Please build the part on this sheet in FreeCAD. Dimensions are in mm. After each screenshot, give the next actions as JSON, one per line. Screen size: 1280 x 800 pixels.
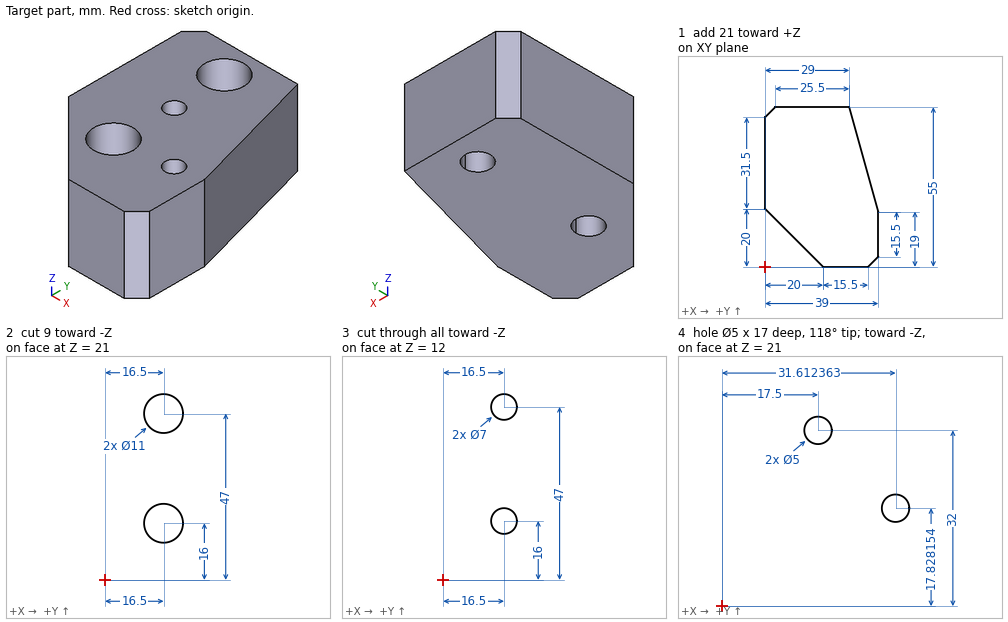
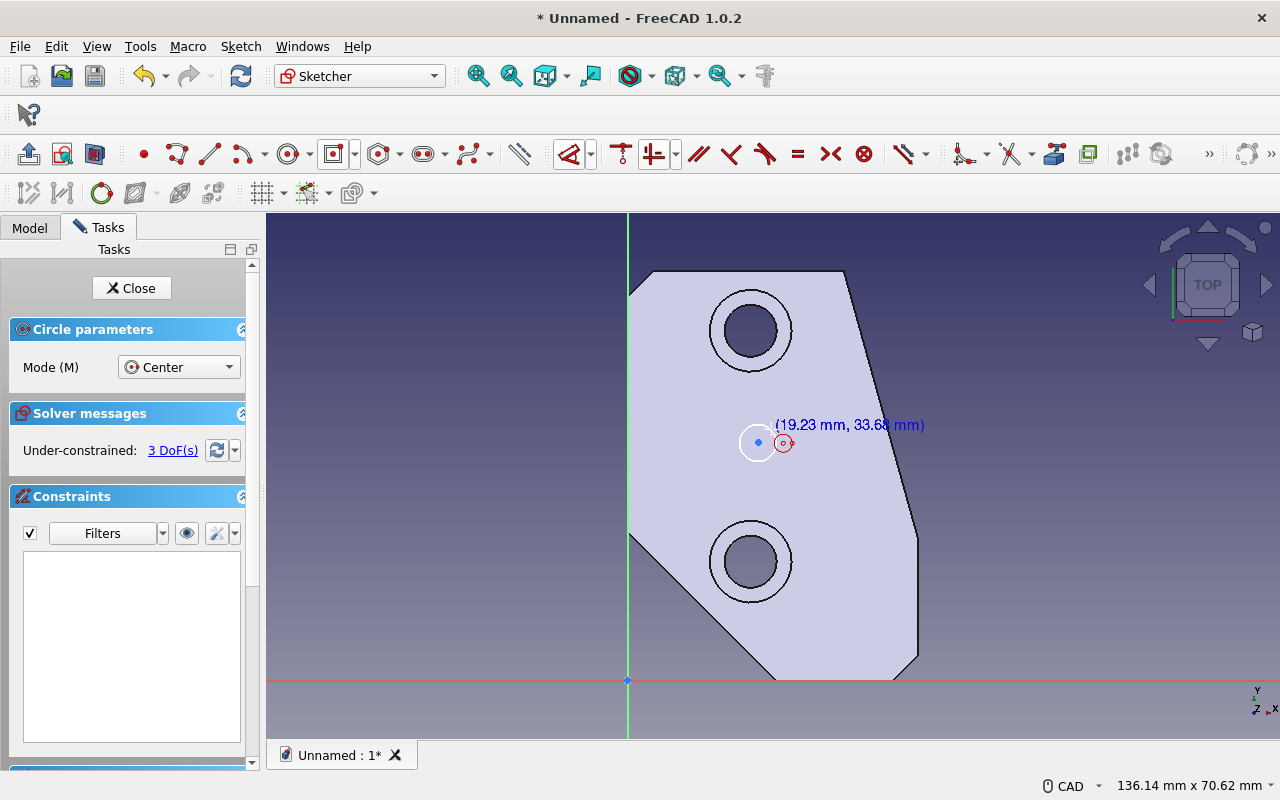
{"action": "left_click", "coordinate": [863, 548]}
{"action": "left_click", "coordinate": [876, 535]}
{"action": "key", "text": "Escape"}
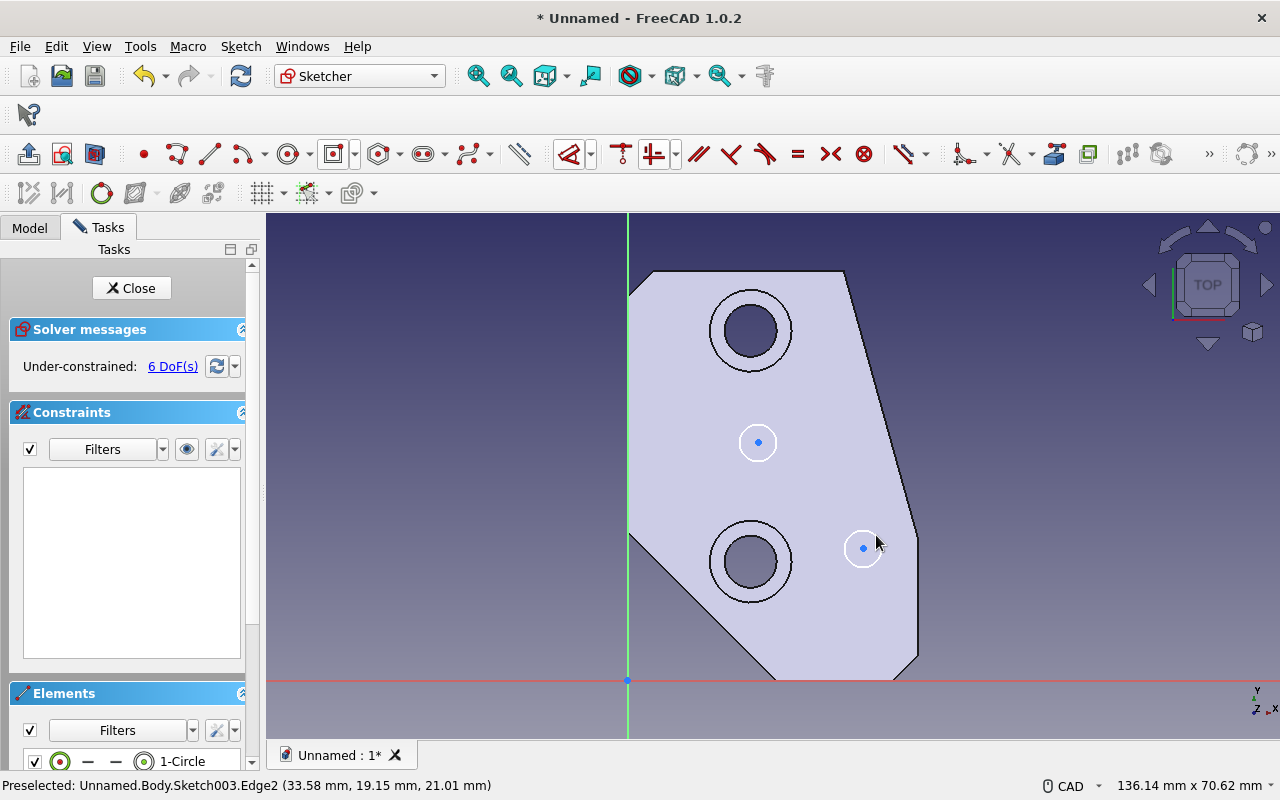
{"action": "left_click", "coordinate": [771, 430]}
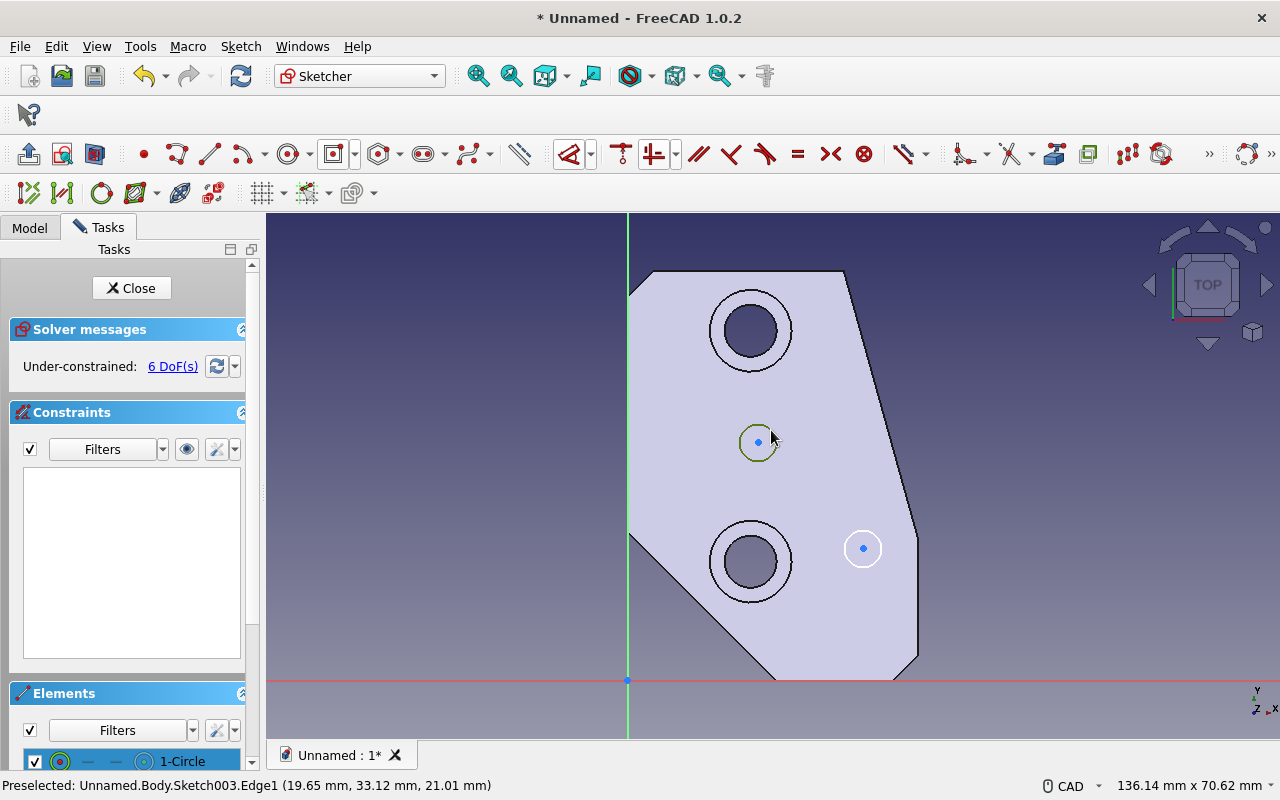
{"action": "left_click", "coordinate": [876, 536]}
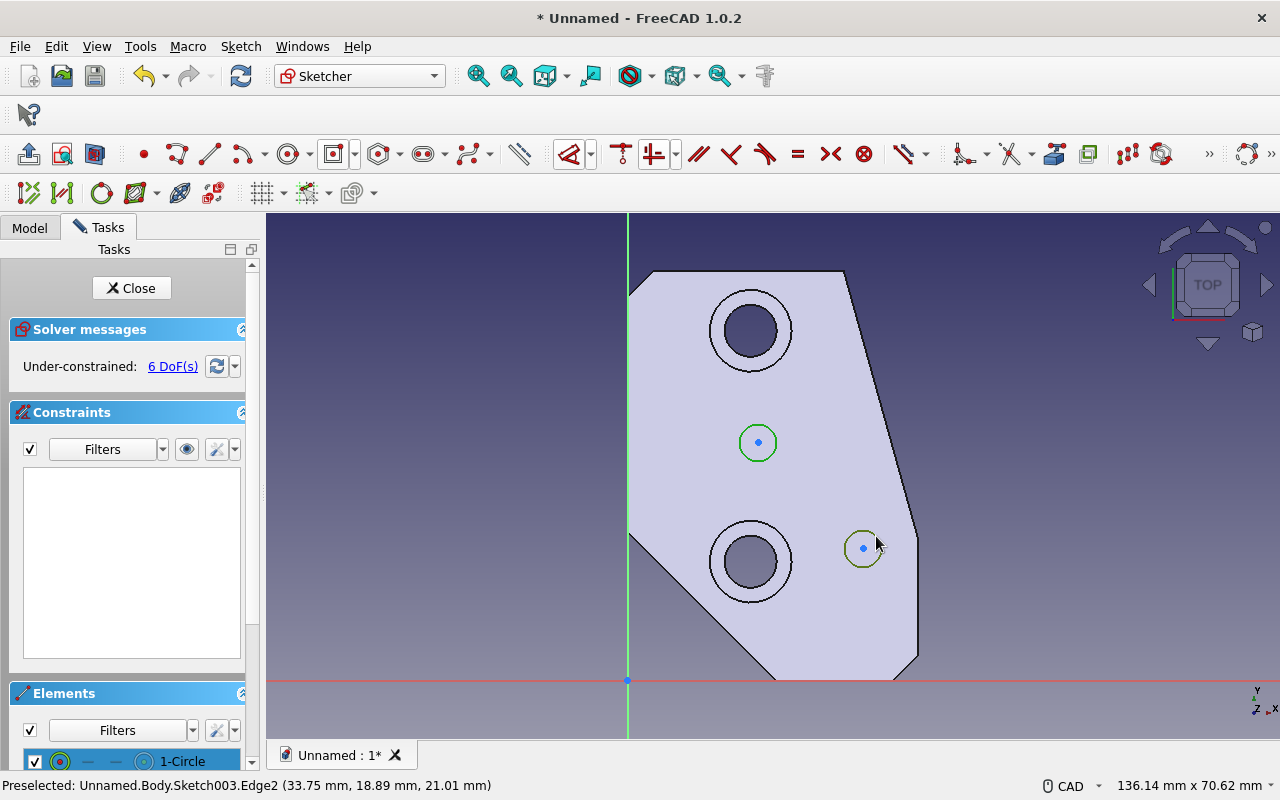
{"action": "left_click", "coordinate": [798, 154]}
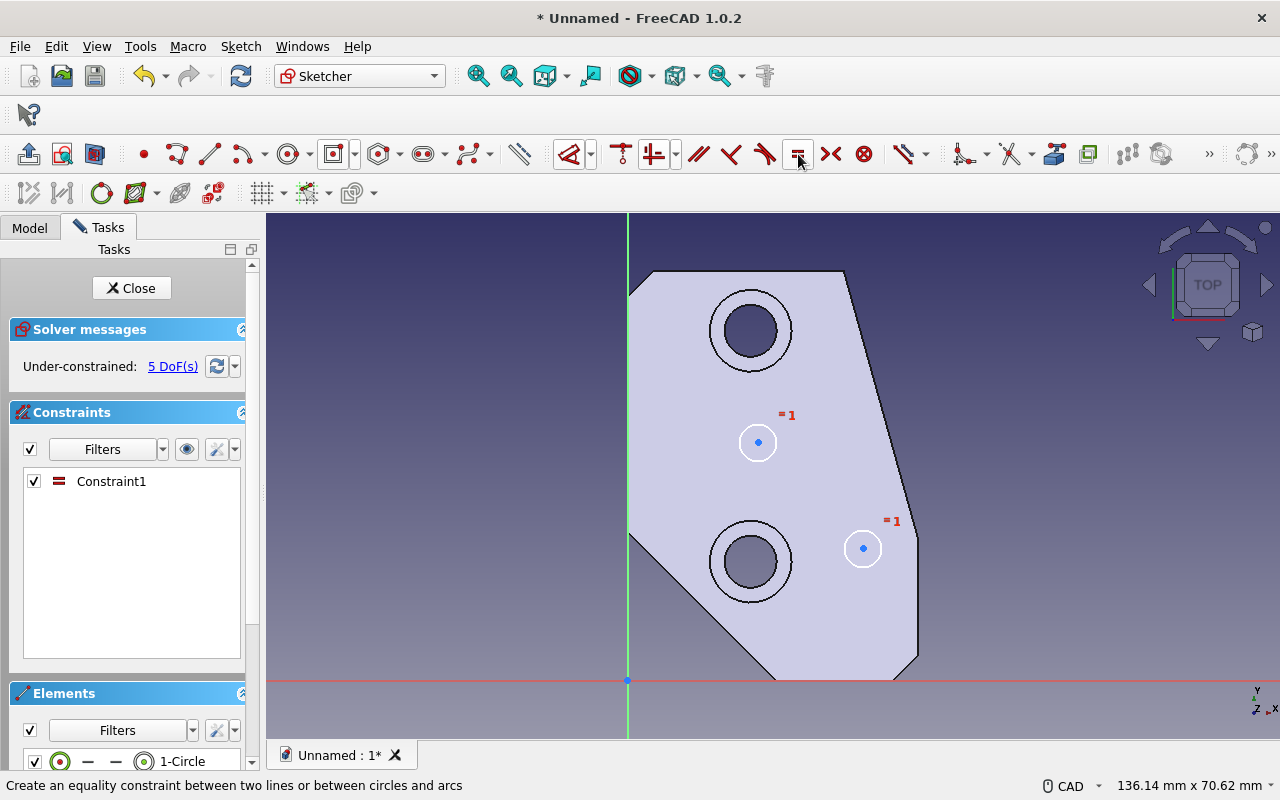
{"action": "left_click", "coordinate": [771, 430]}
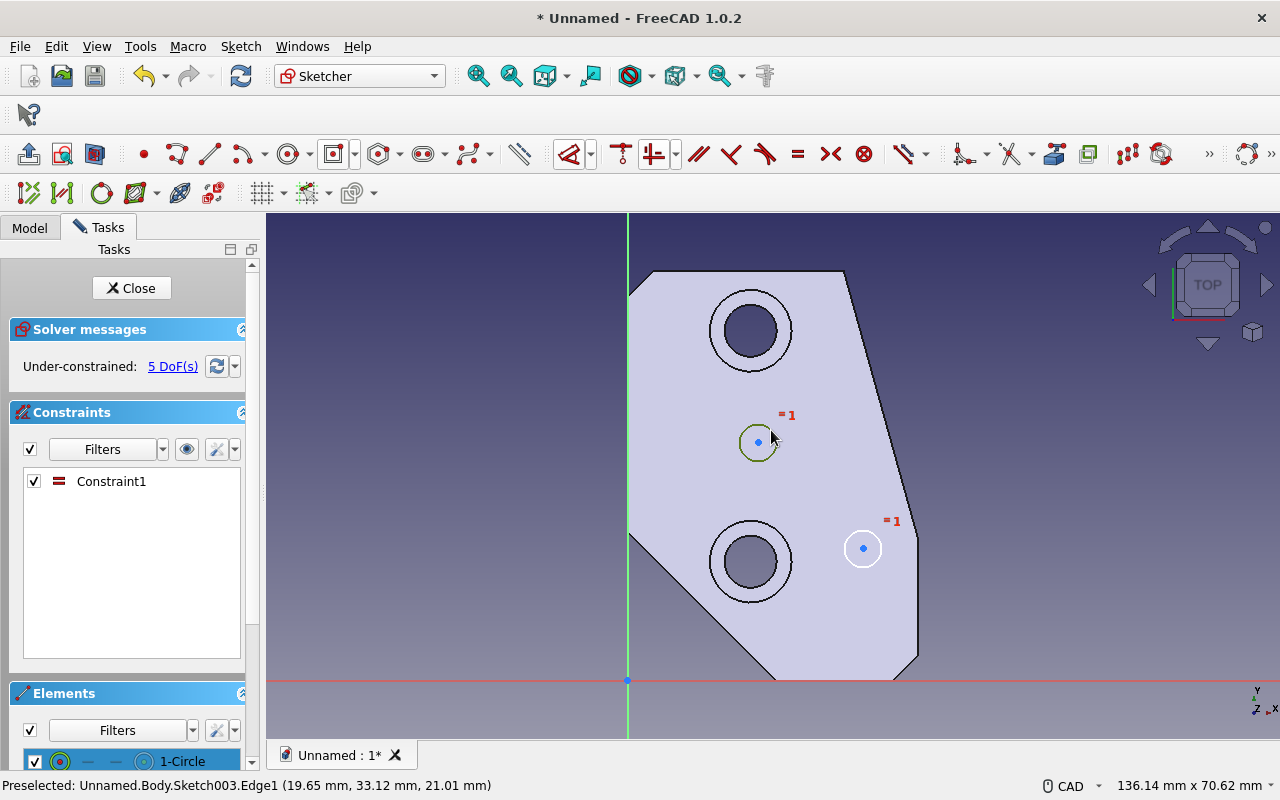
{"action": "left_click", "coordinate": [590, 154]}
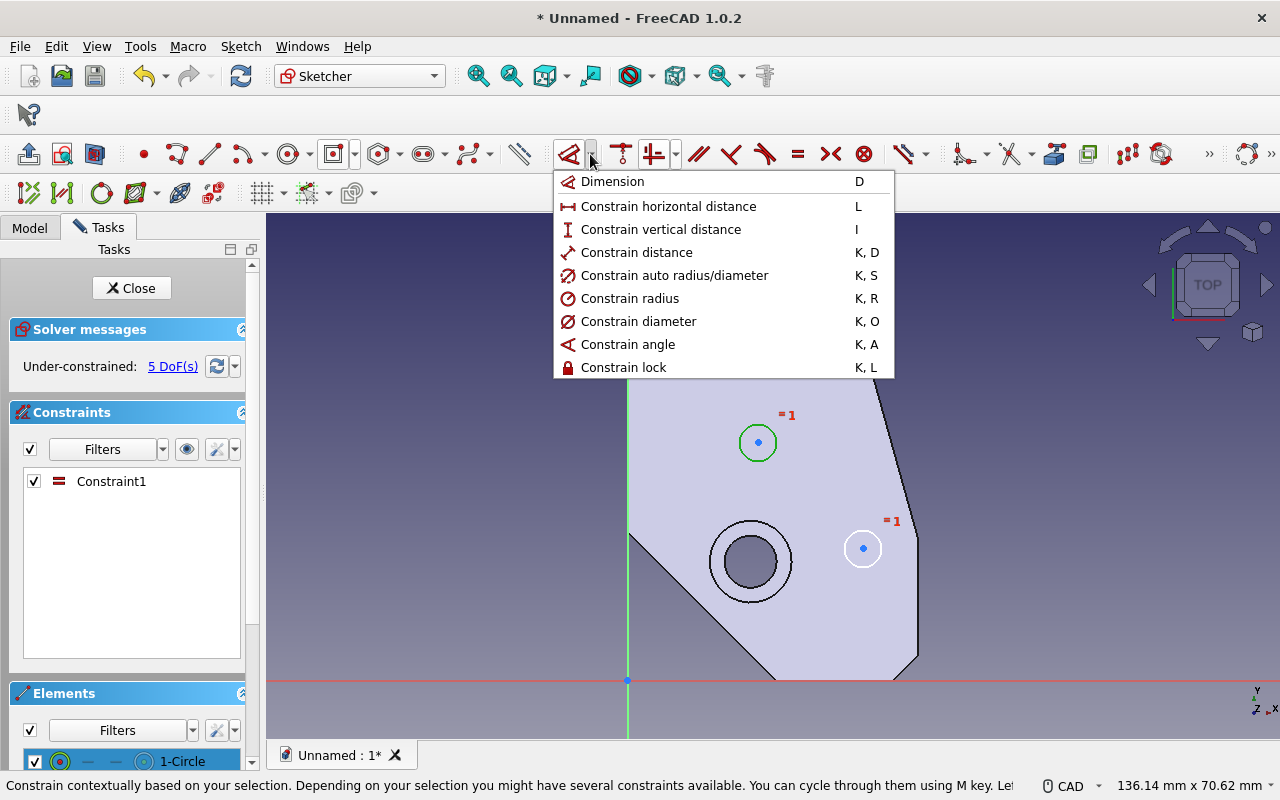
{"action": "left_click", "coordinate": [724, 322]}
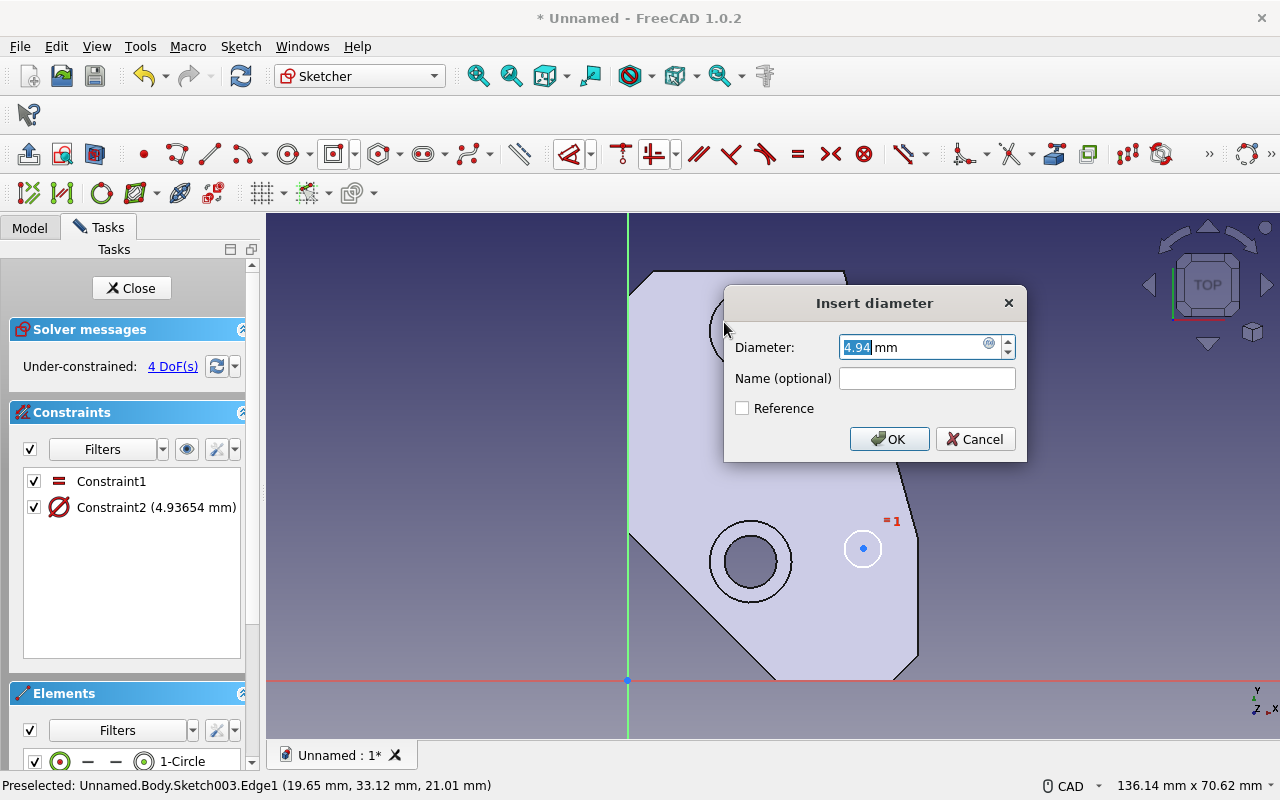
{"action": "type", "text": "5"}
{"action": "key", "text": "Return"}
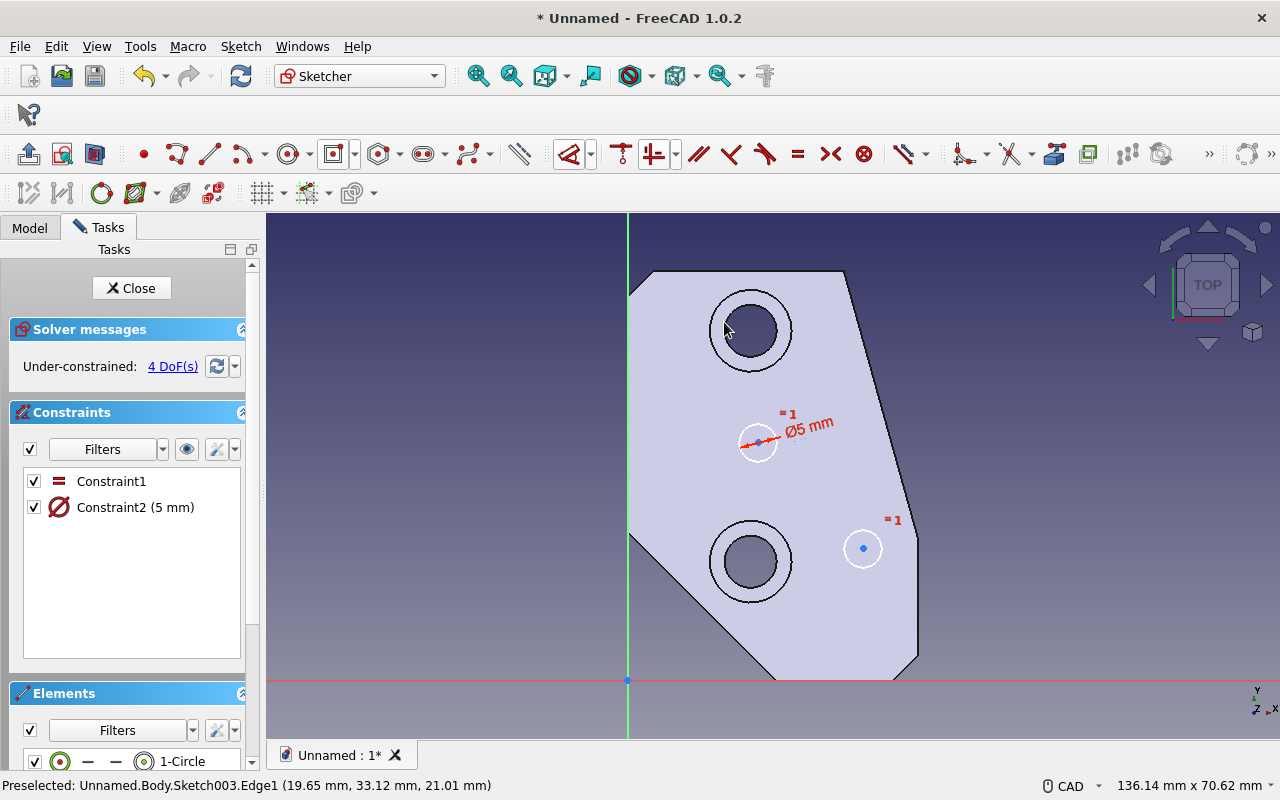
{"action": "left_click", "coordinate": [758, 443]}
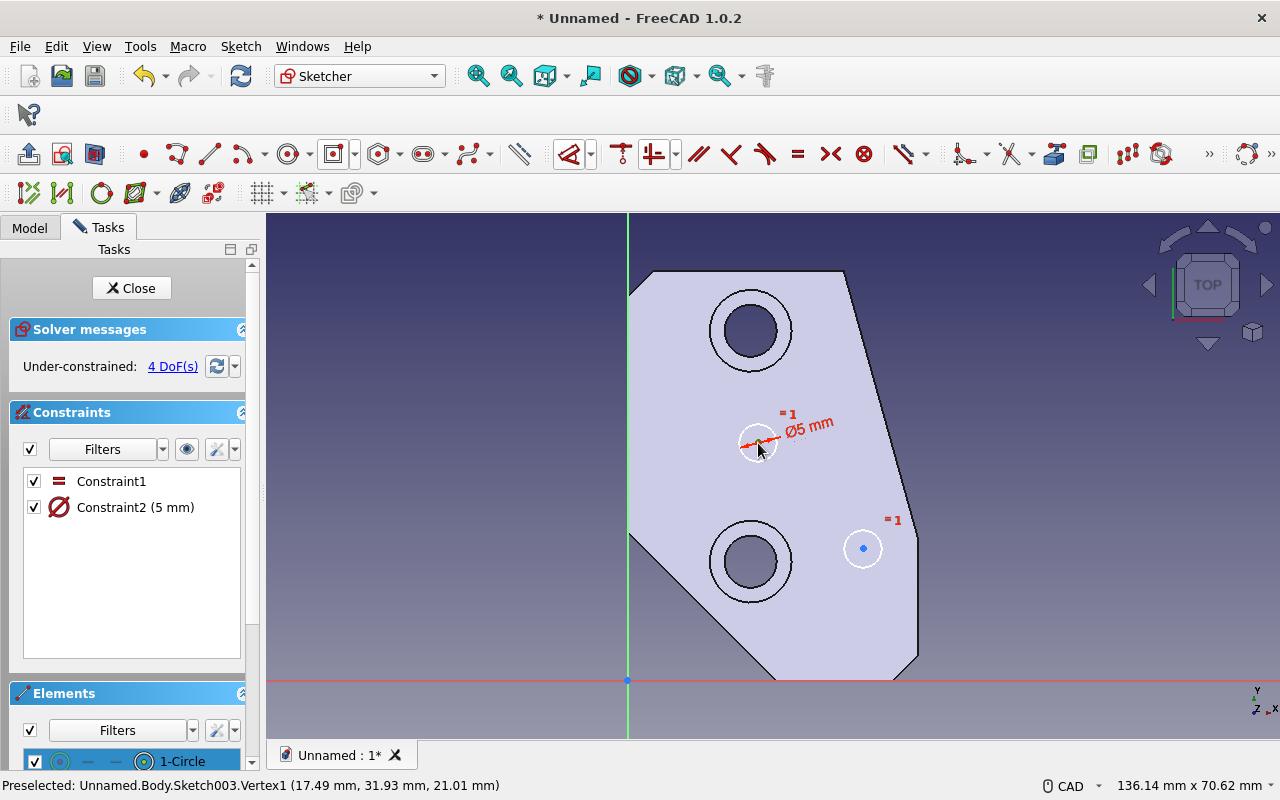
{"action": "left_click", "coordinate": [590, 154]}